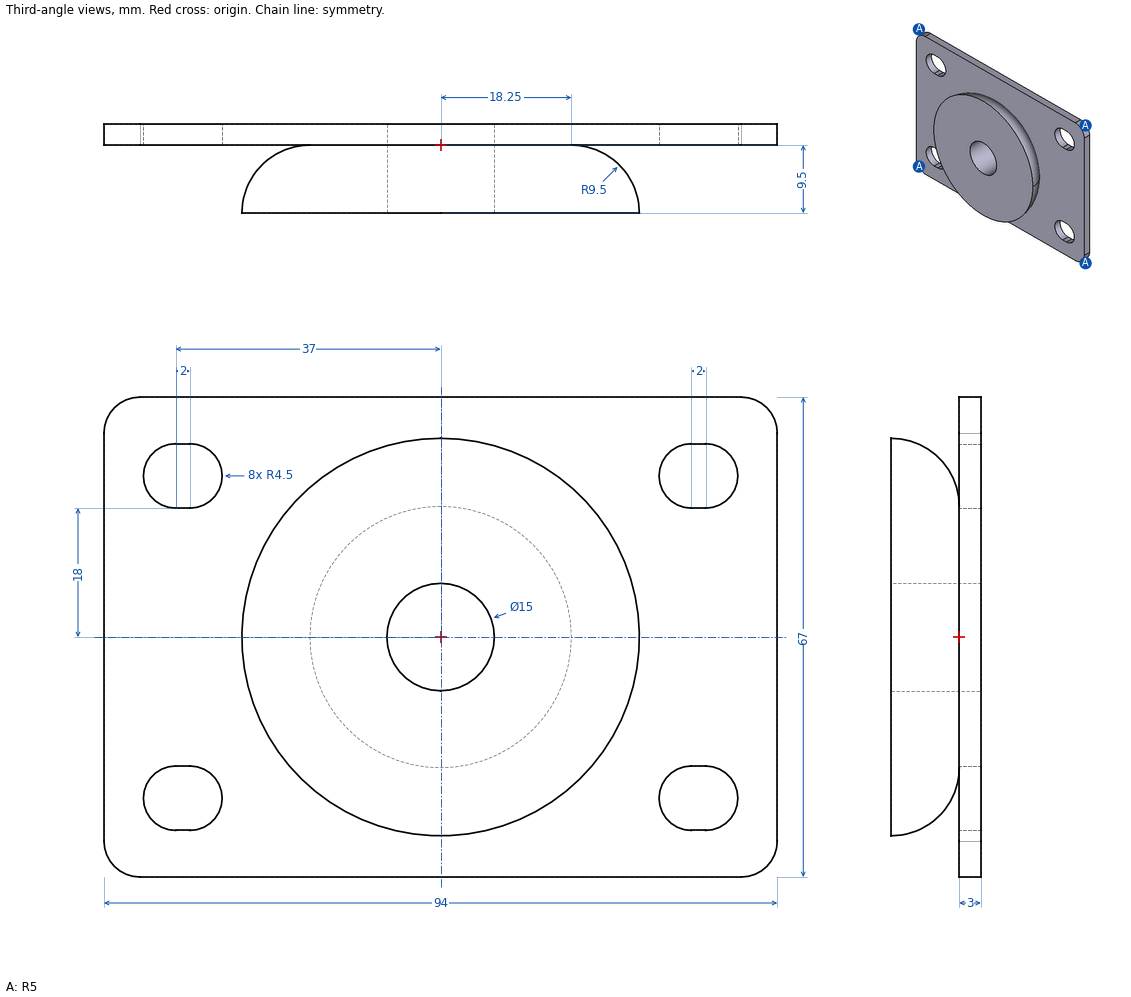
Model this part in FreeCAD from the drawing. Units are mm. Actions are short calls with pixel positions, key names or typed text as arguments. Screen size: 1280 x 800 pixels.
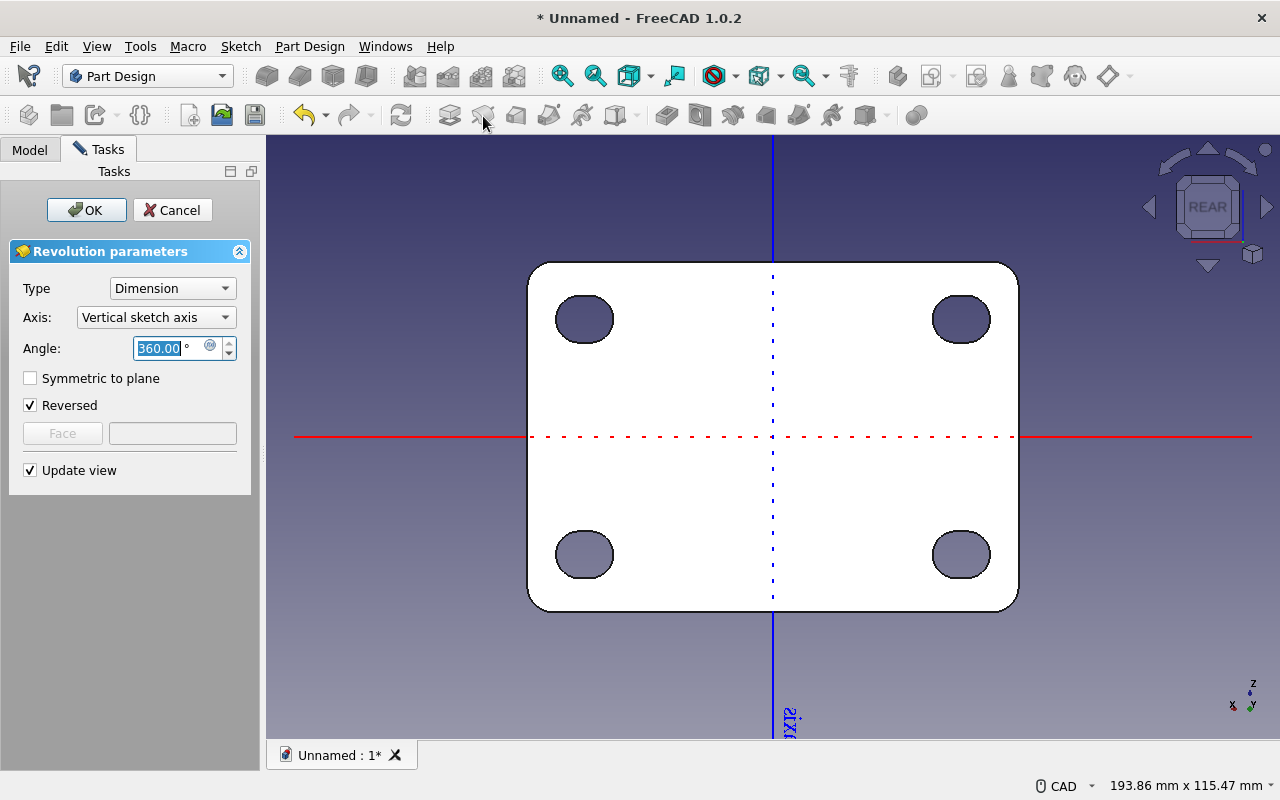
click(87, 210)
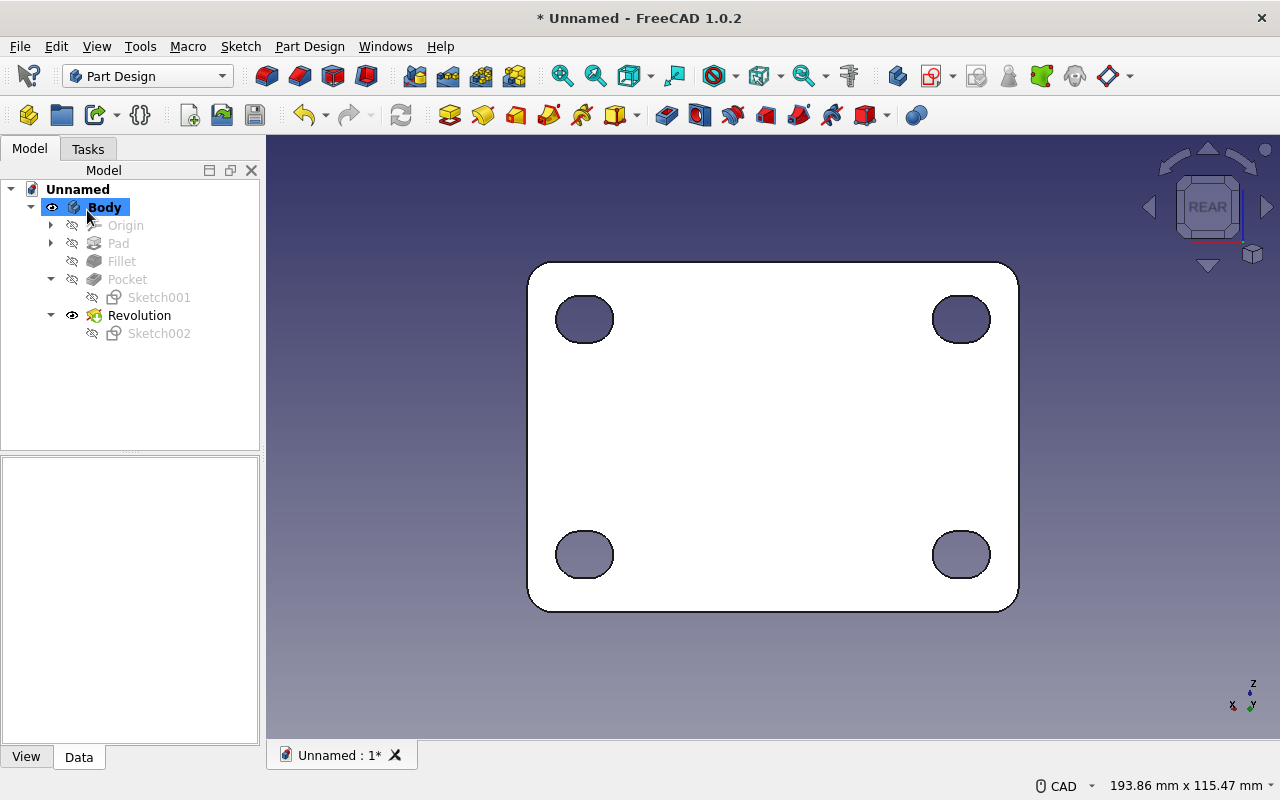
key(0)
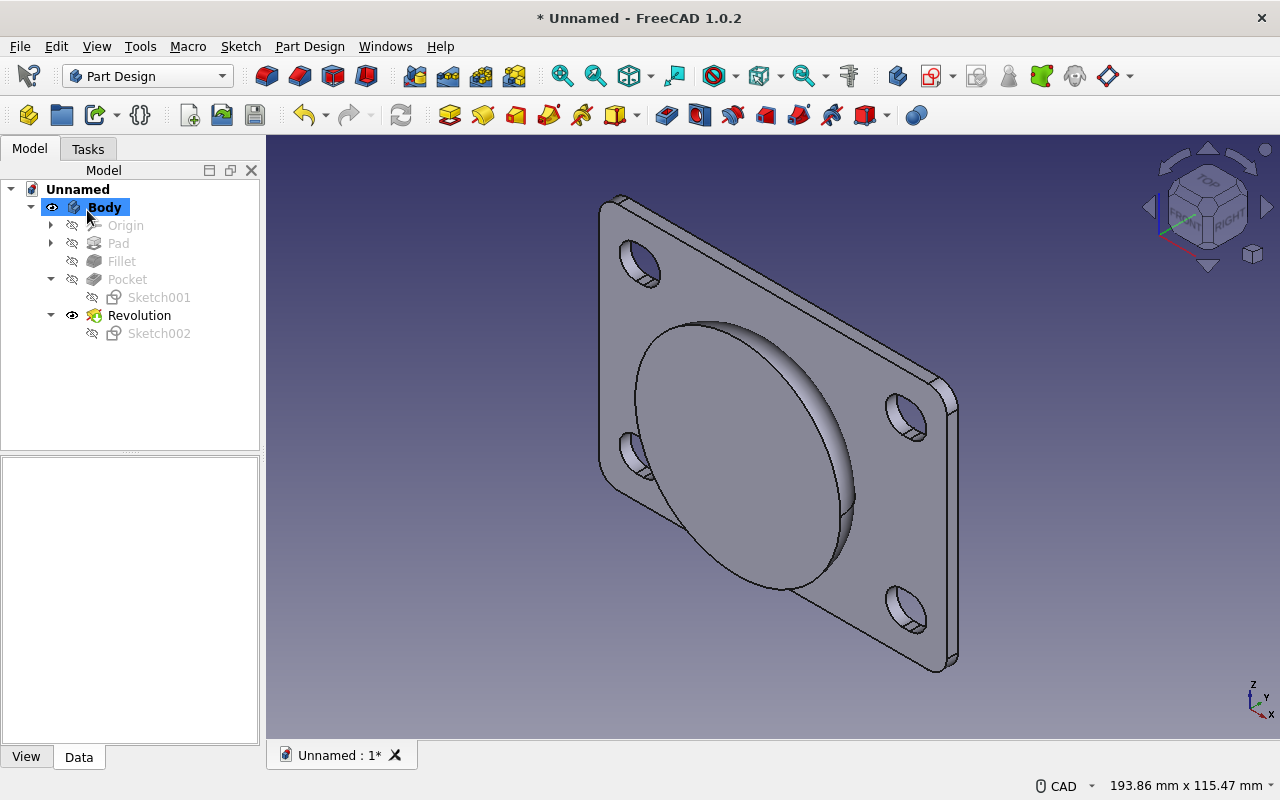
click(738, 456)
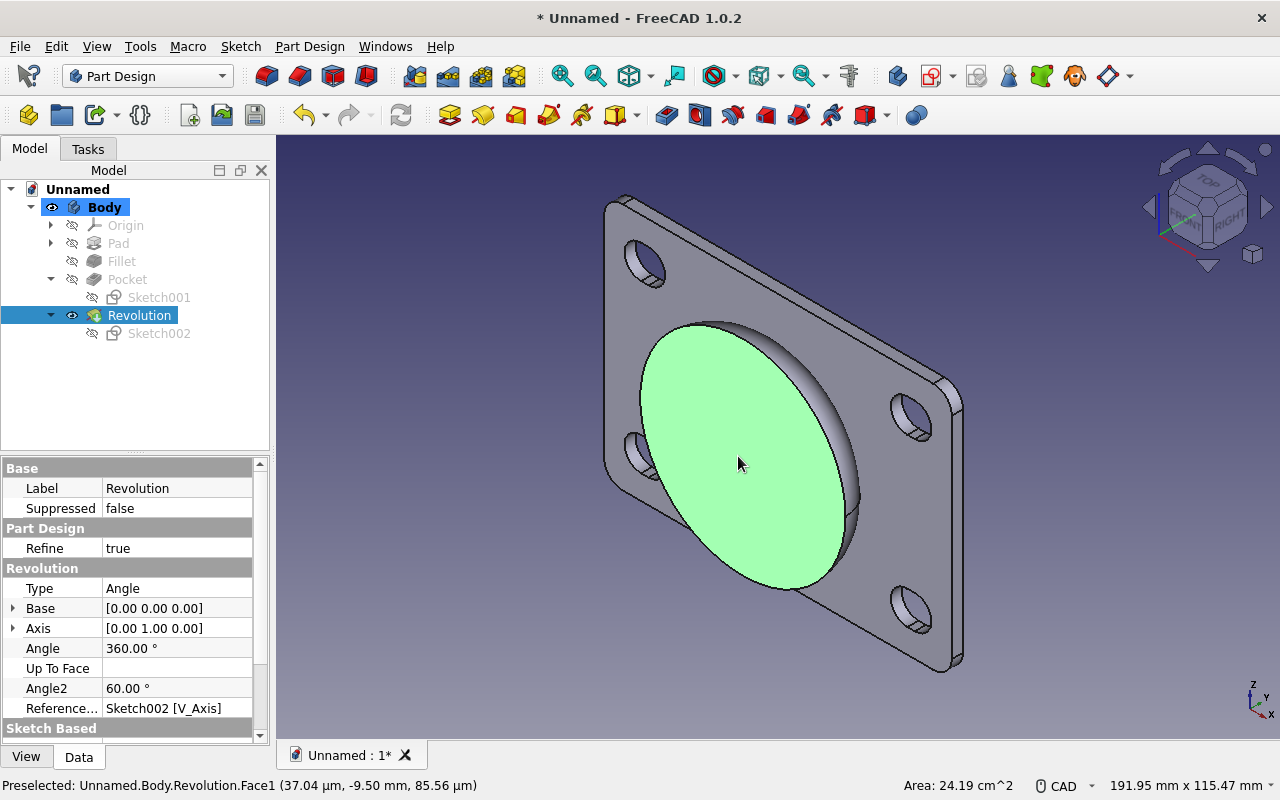
click(930, 76)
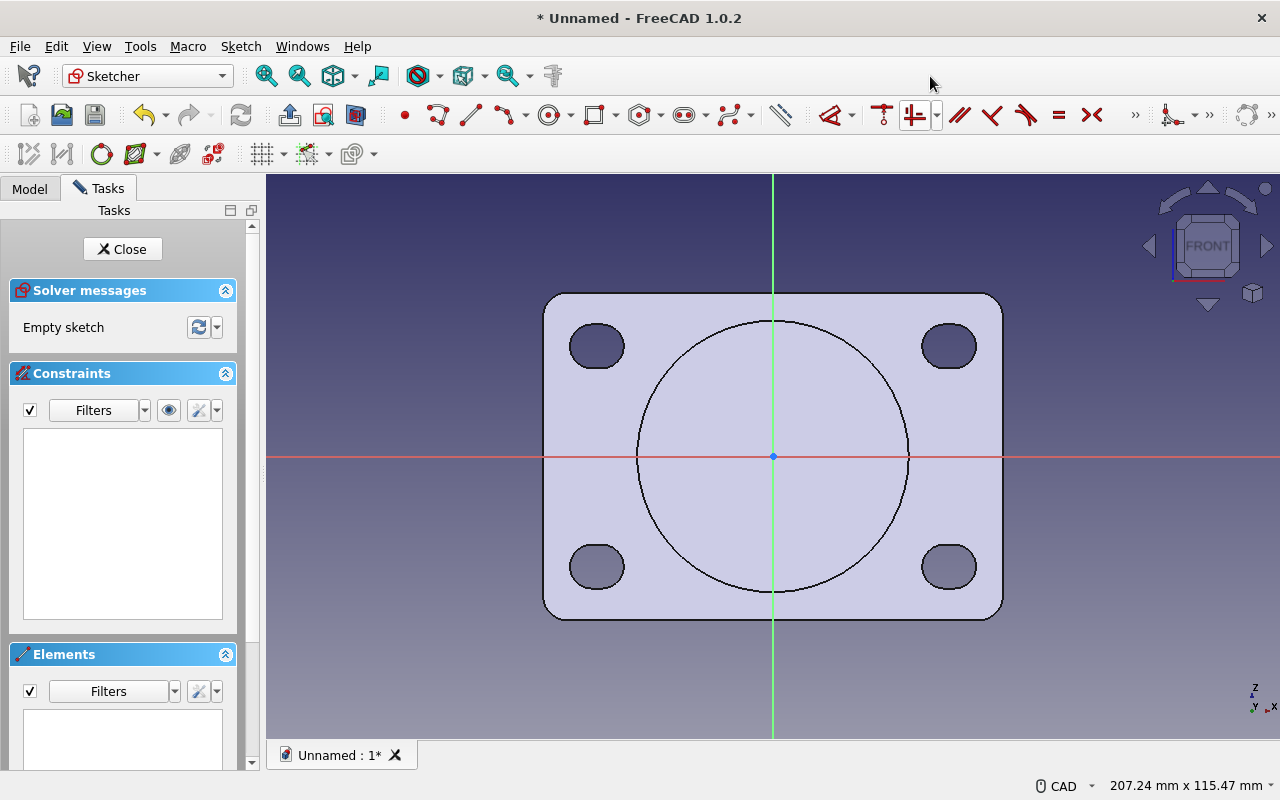
scroll(790, 457, up, 8)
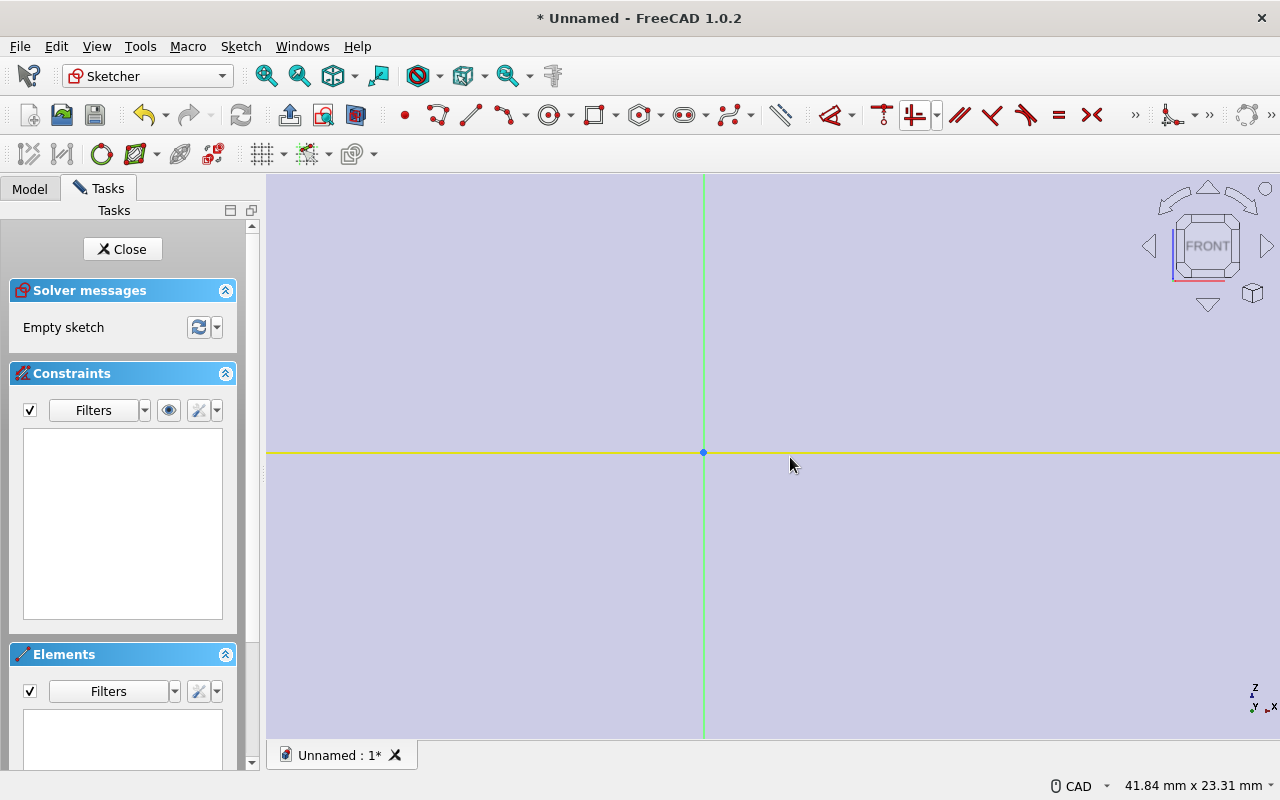
key(g)
key(c)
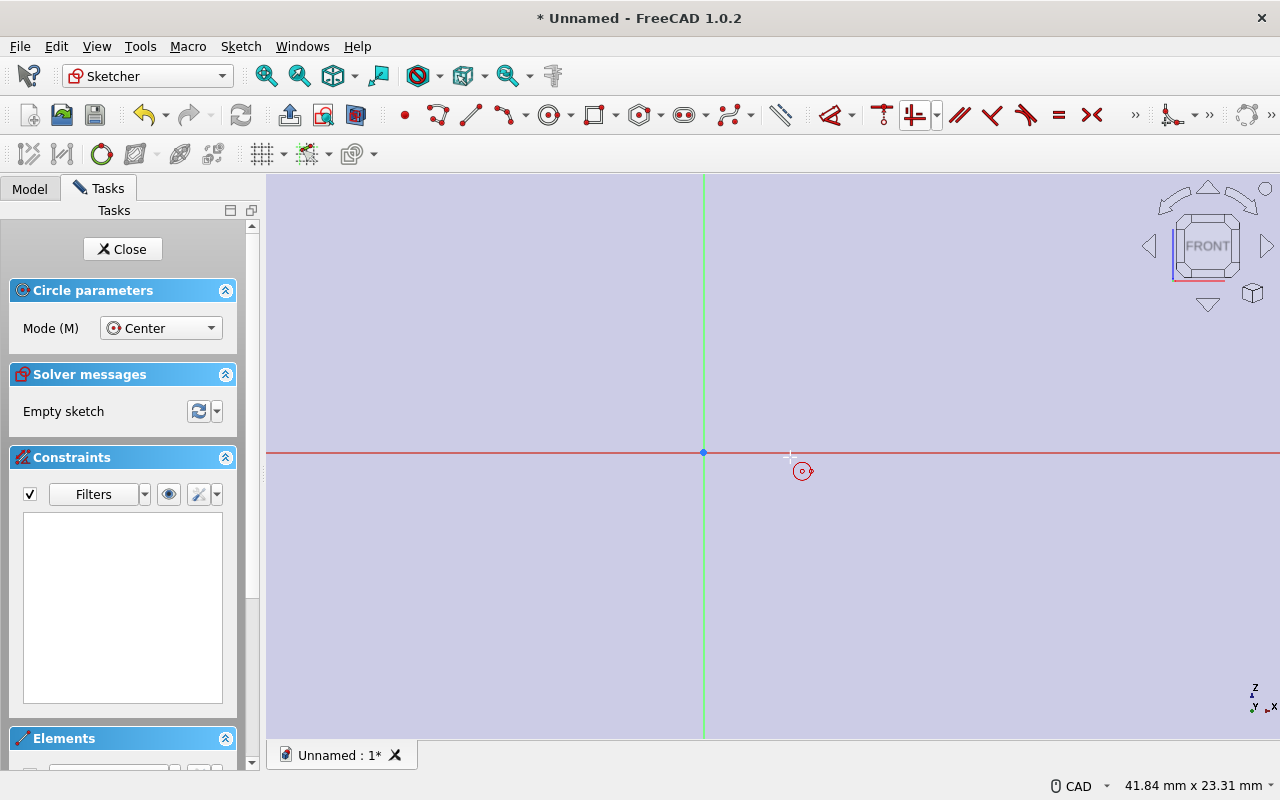
click(704, 453)
move(832, 324)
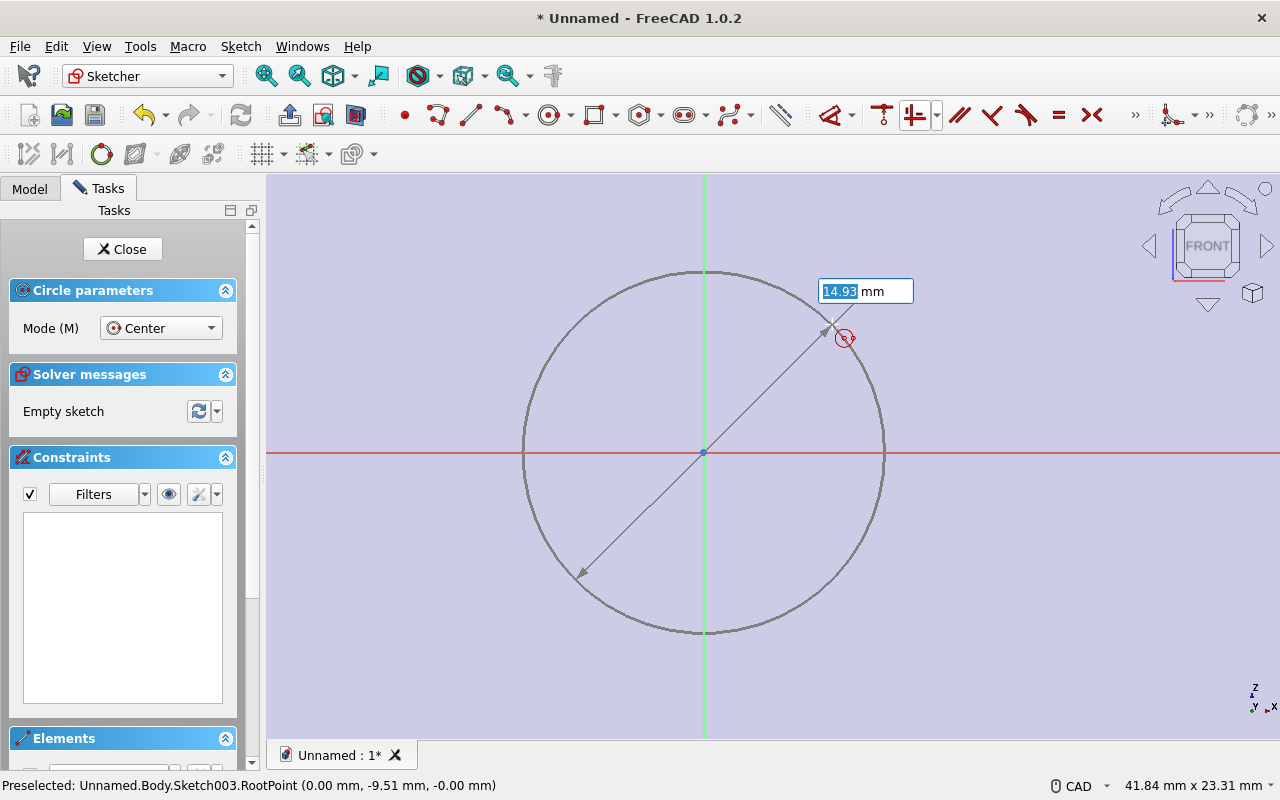
text(15)
key(Return)
key(Escape)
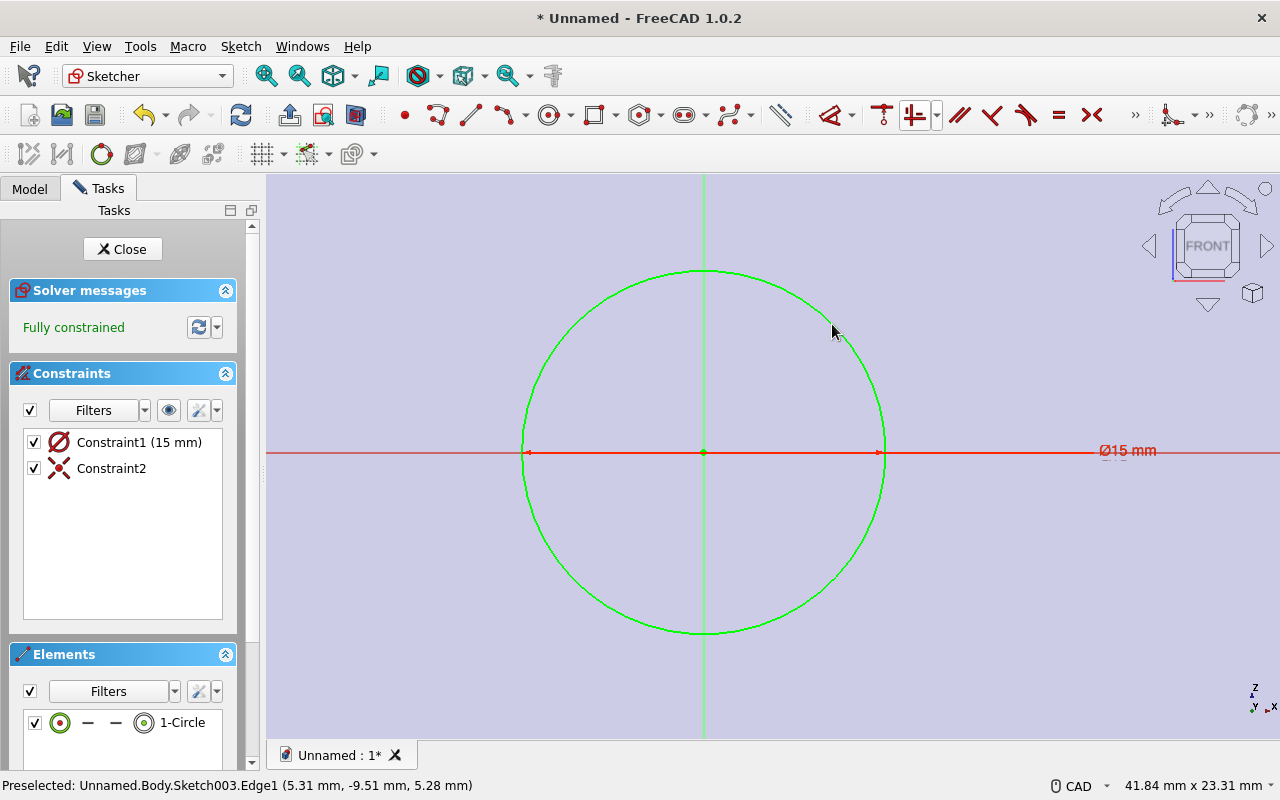
click(123, 249)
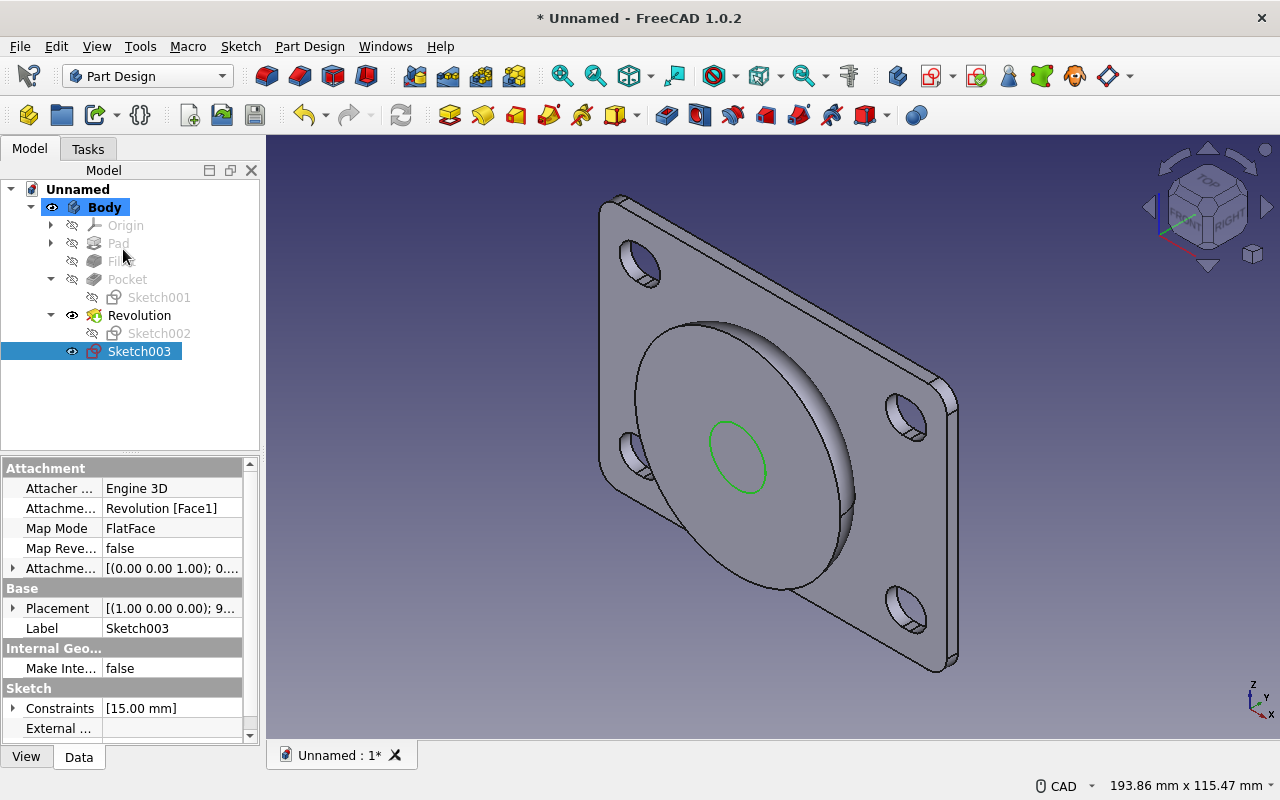
click(667, 116)